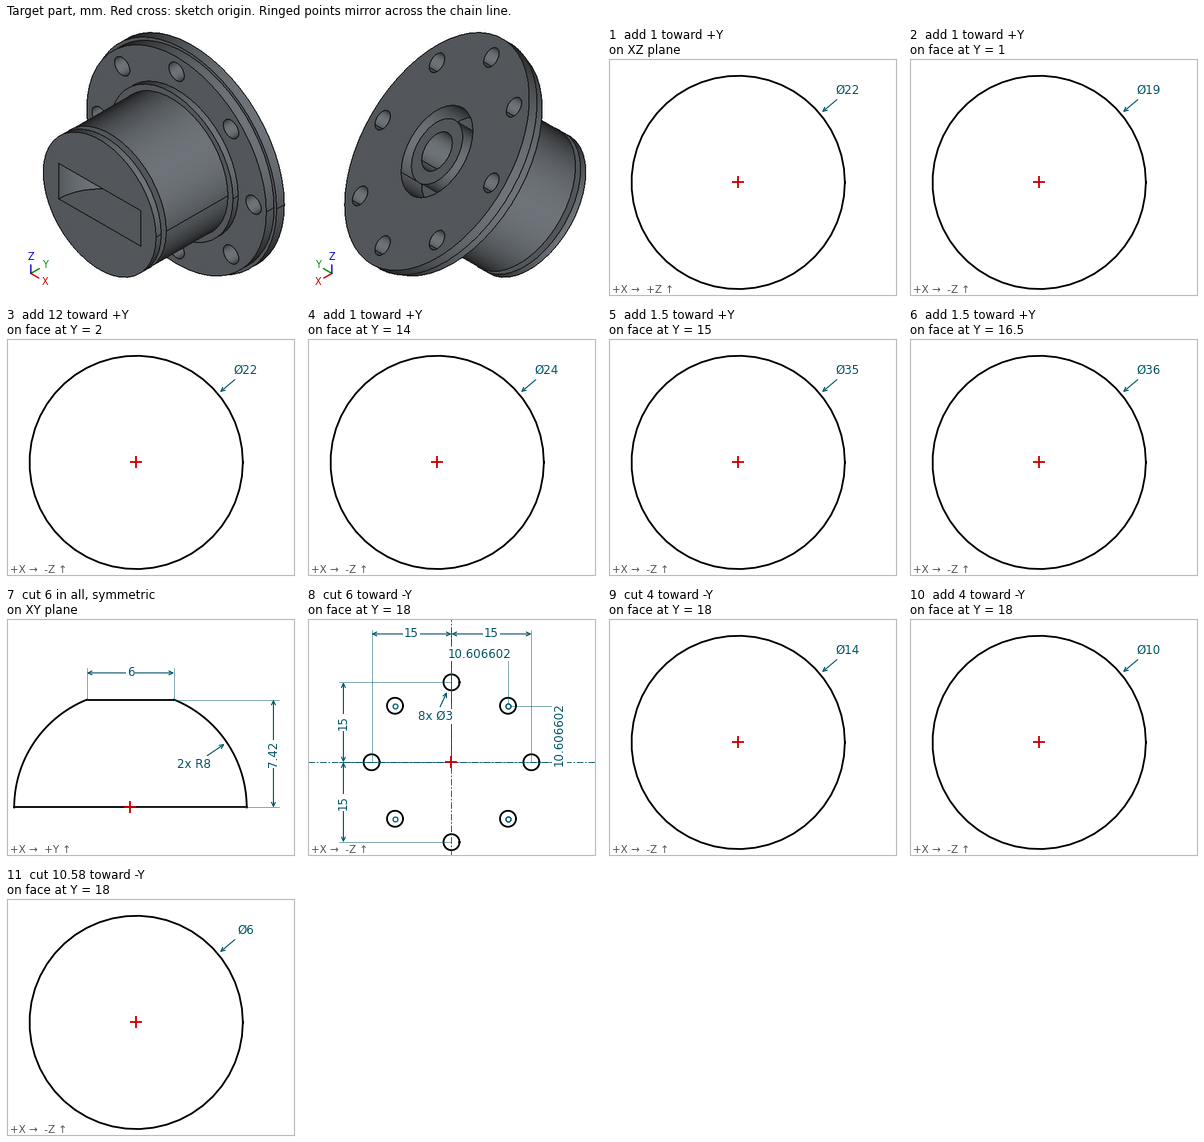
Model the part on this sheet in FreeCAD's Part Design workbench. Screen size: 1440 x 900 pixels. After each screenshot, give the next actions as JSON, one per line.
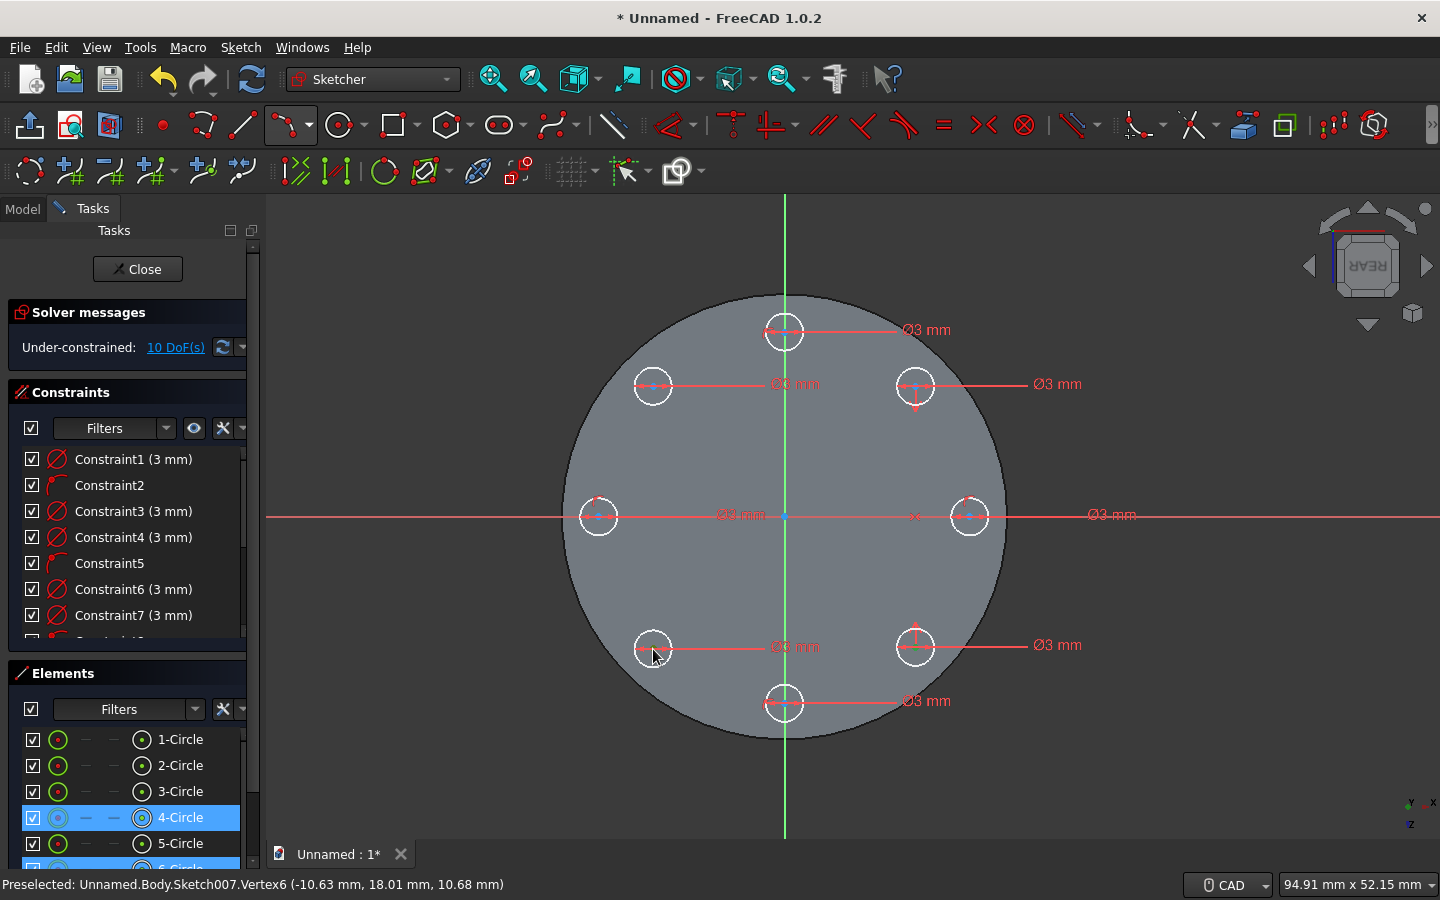
{"action": "left_click", "coordinate": [785, 769]}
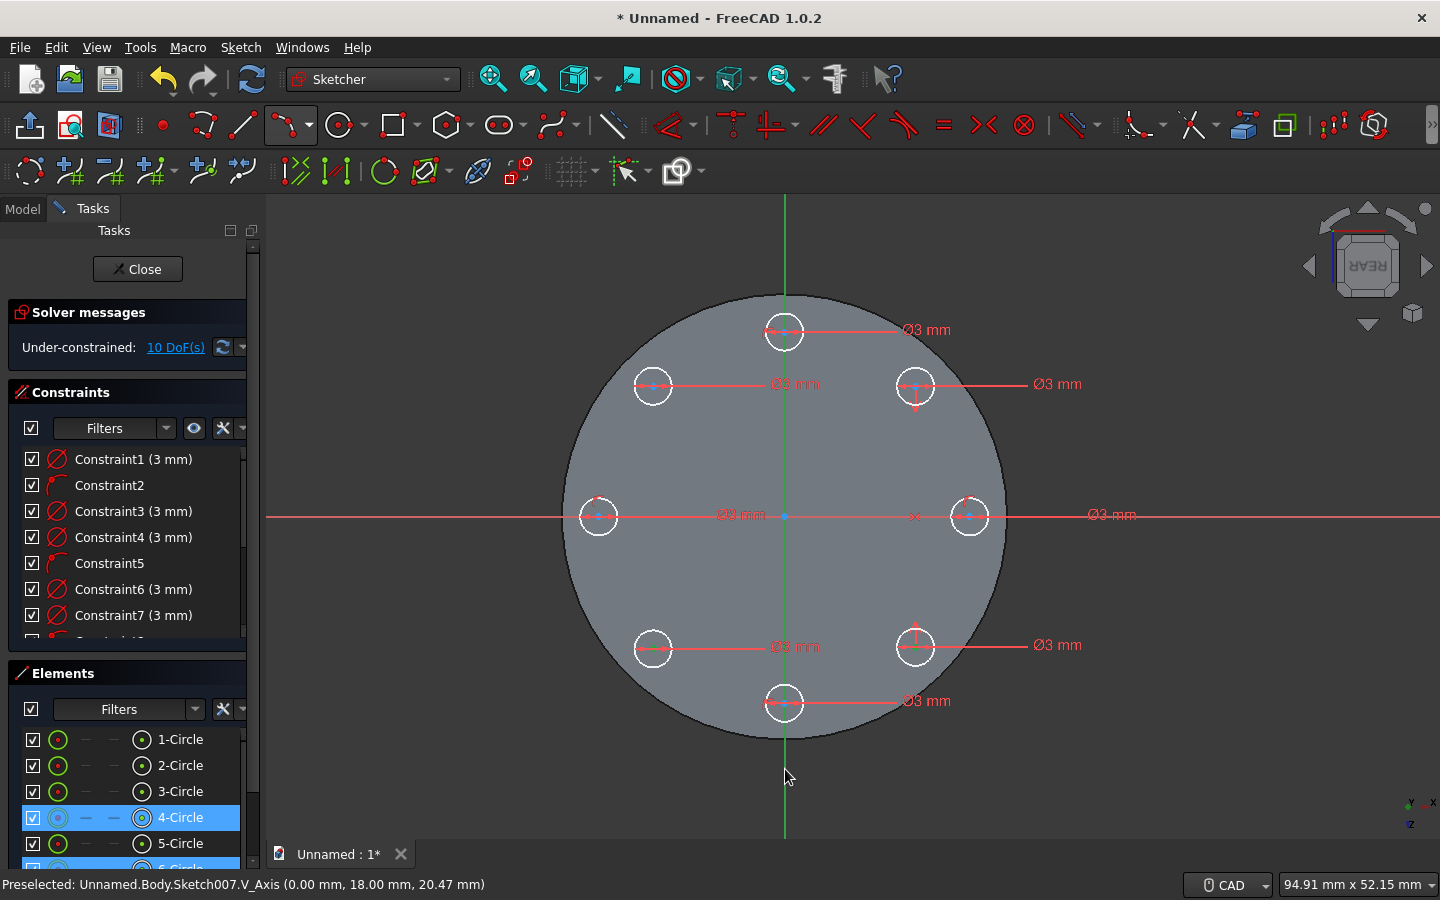
{"action": "left_click", "coordinate": [984, 126]}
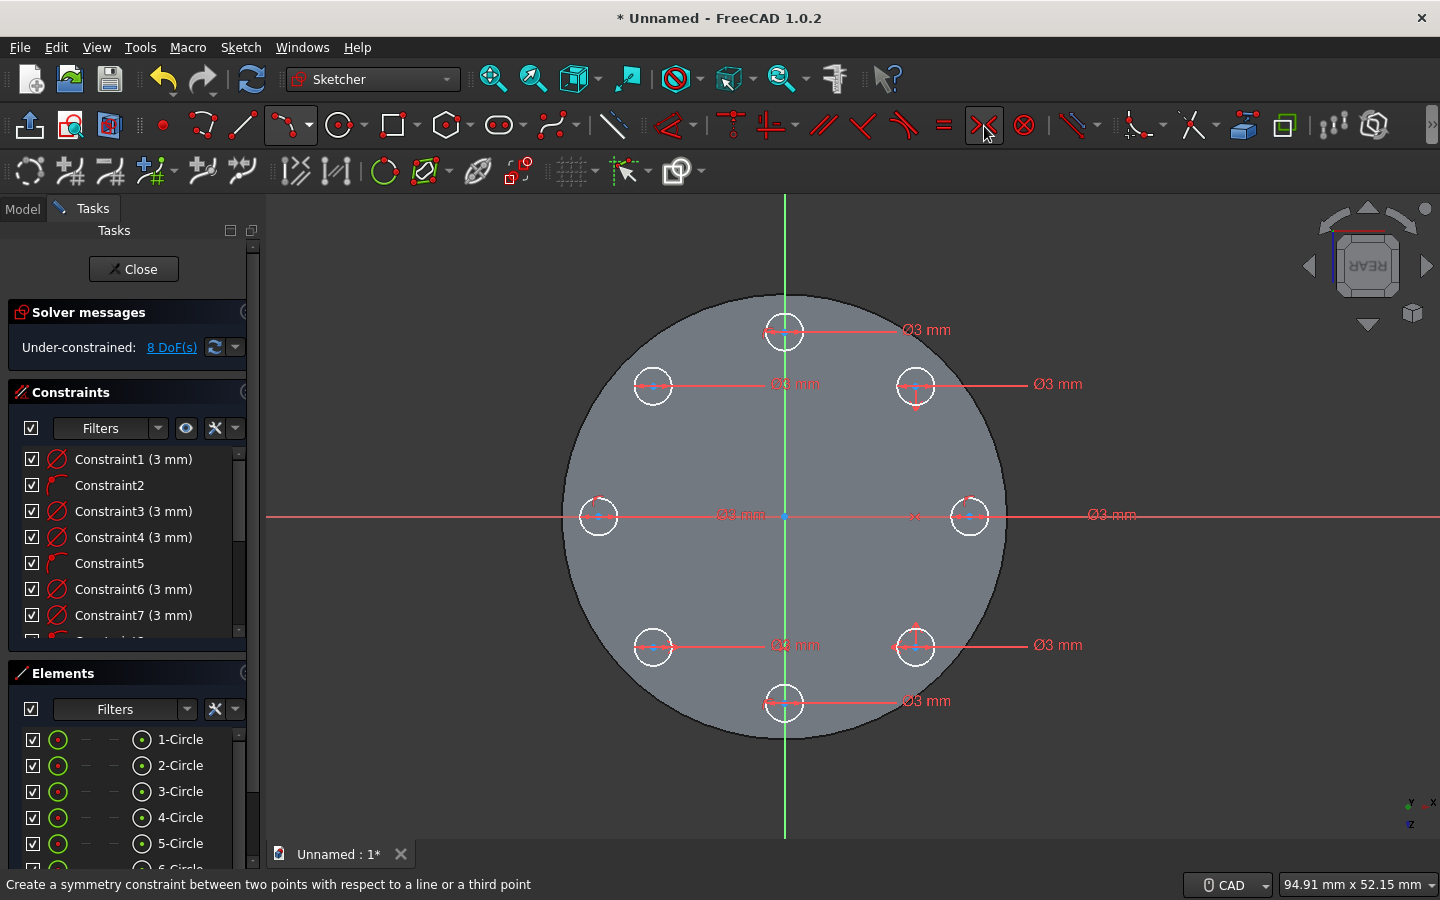
{"action": "left_click", "coordinate": [916, 386]}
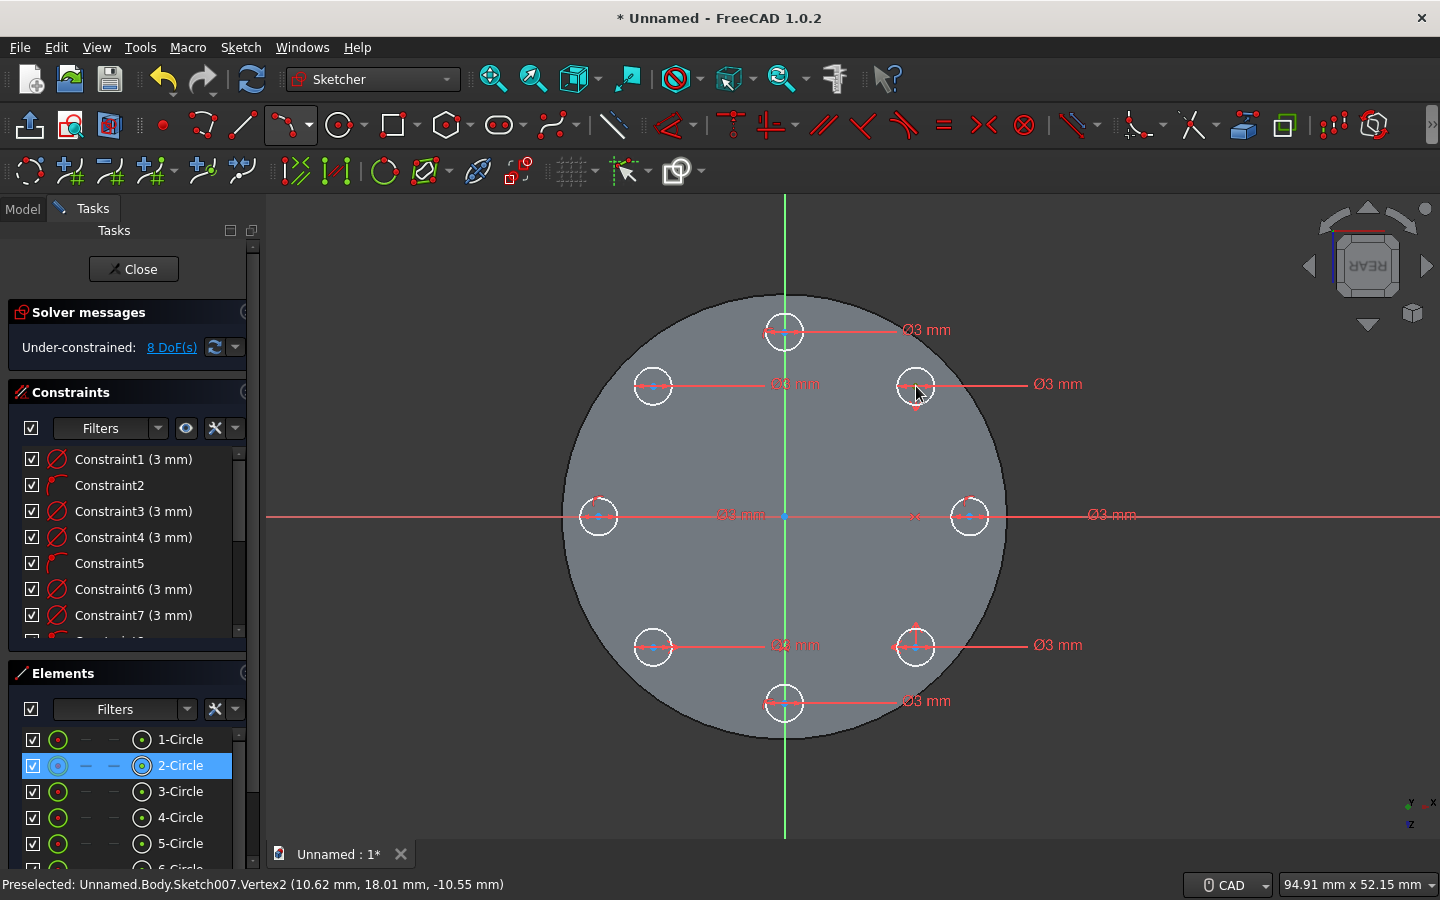
{"action": "left_click", "coordinate": [653, 386]}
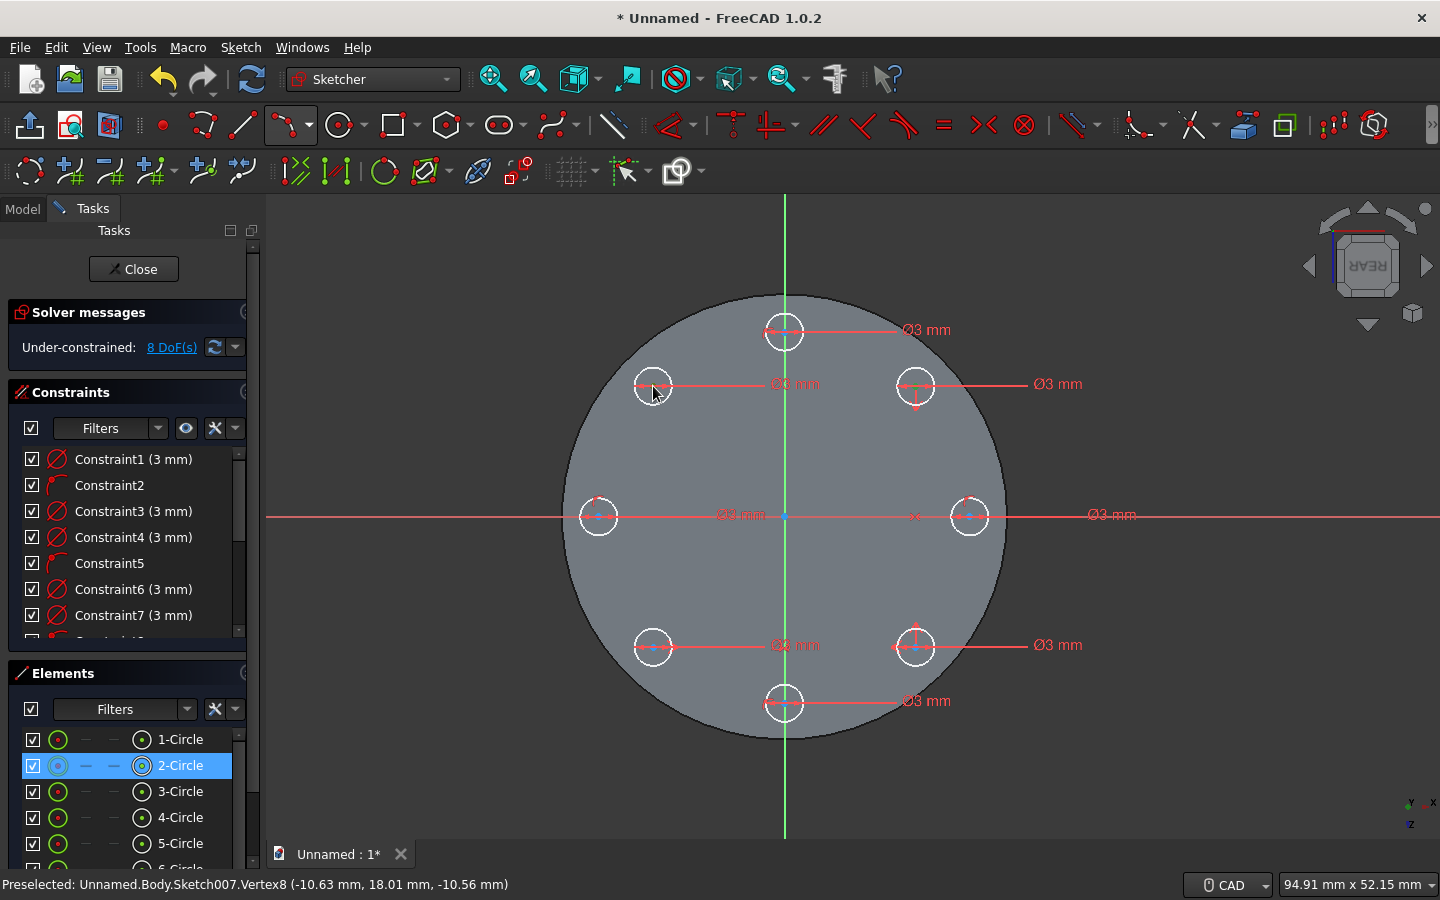
{"action": "left_click", "coordinate": [785, 769]}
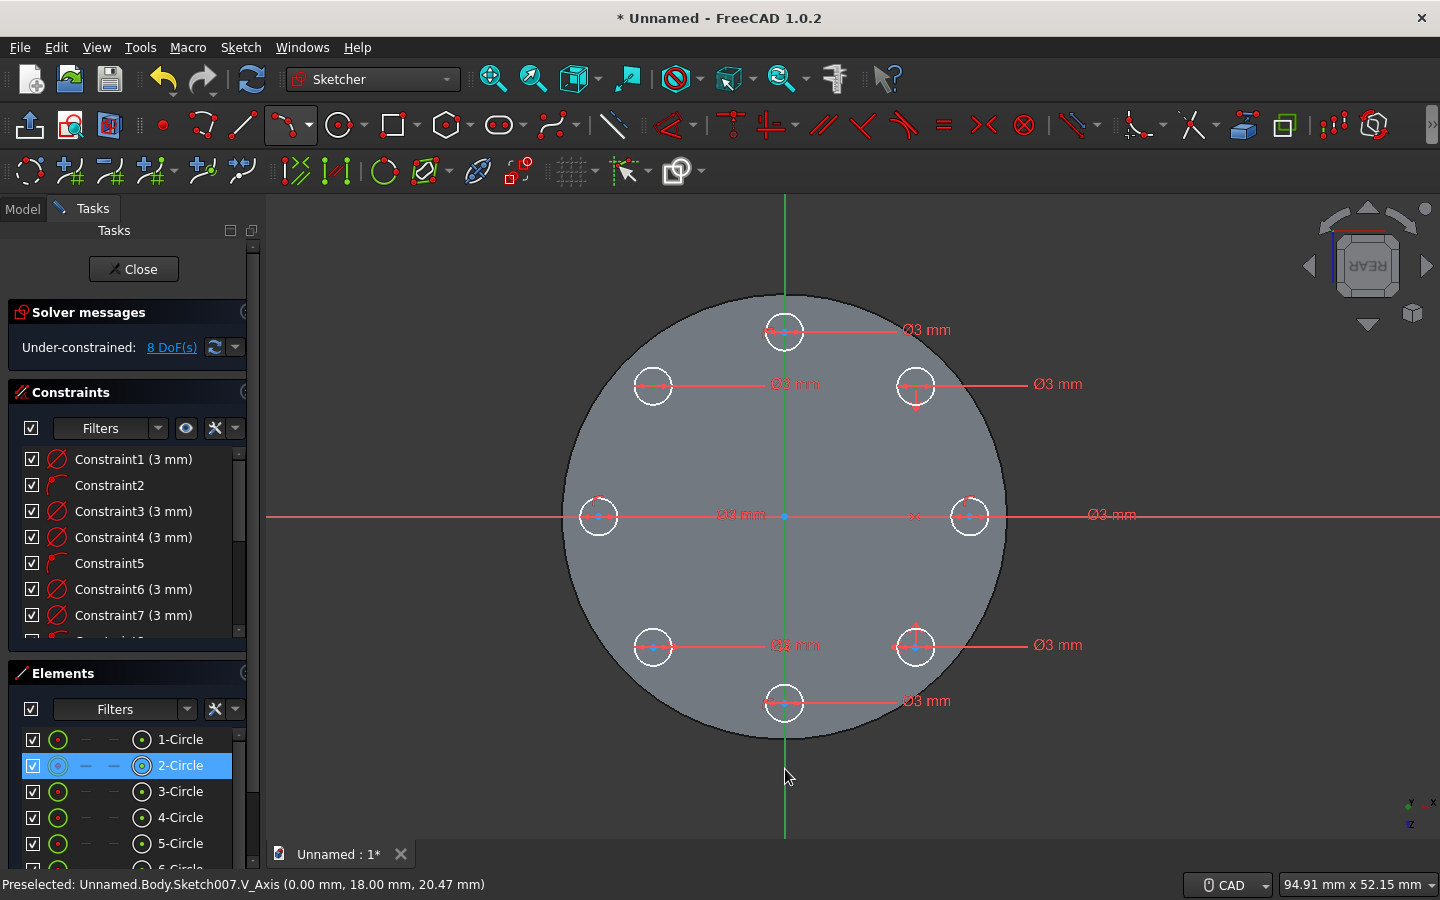
{"action": "left_click", "coordinate": [984, 126]}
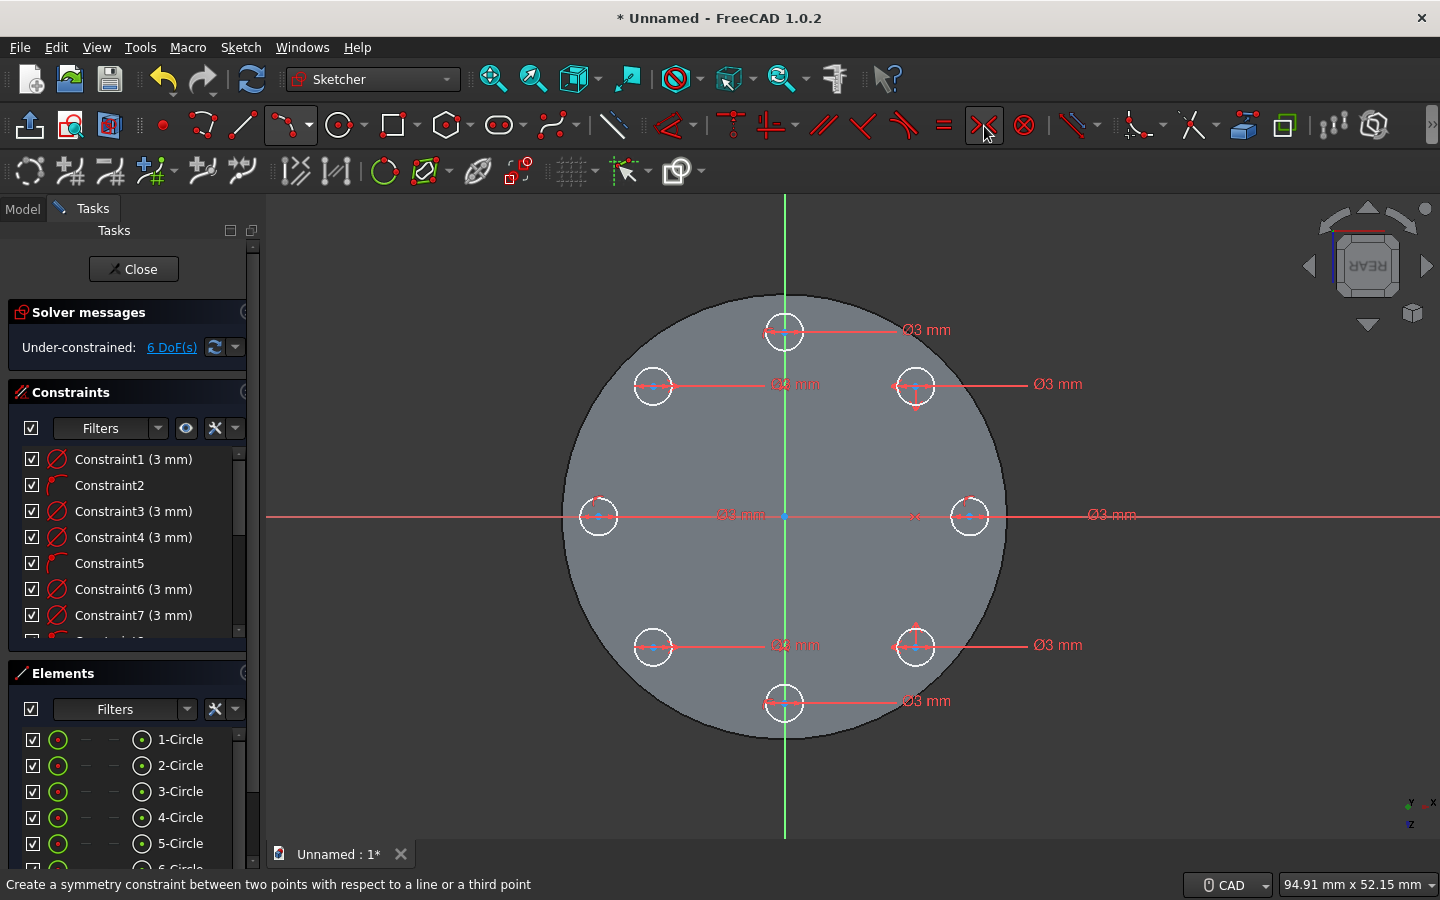
{"action": "left_click", "coordinate": [668, 126]}